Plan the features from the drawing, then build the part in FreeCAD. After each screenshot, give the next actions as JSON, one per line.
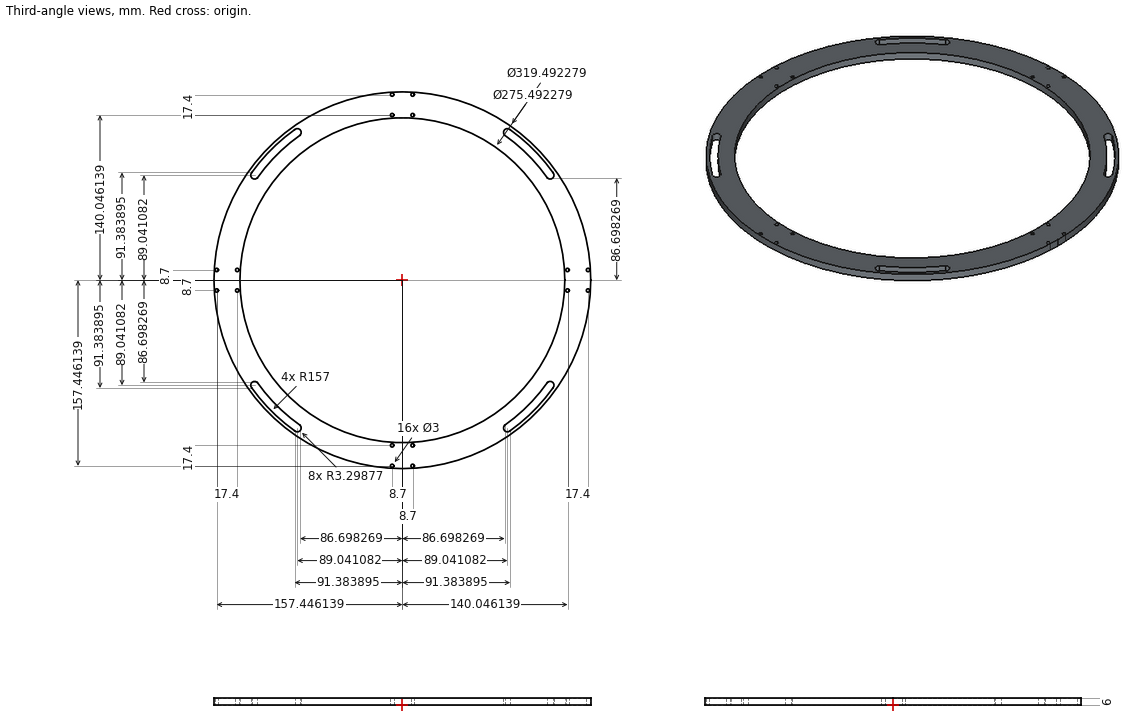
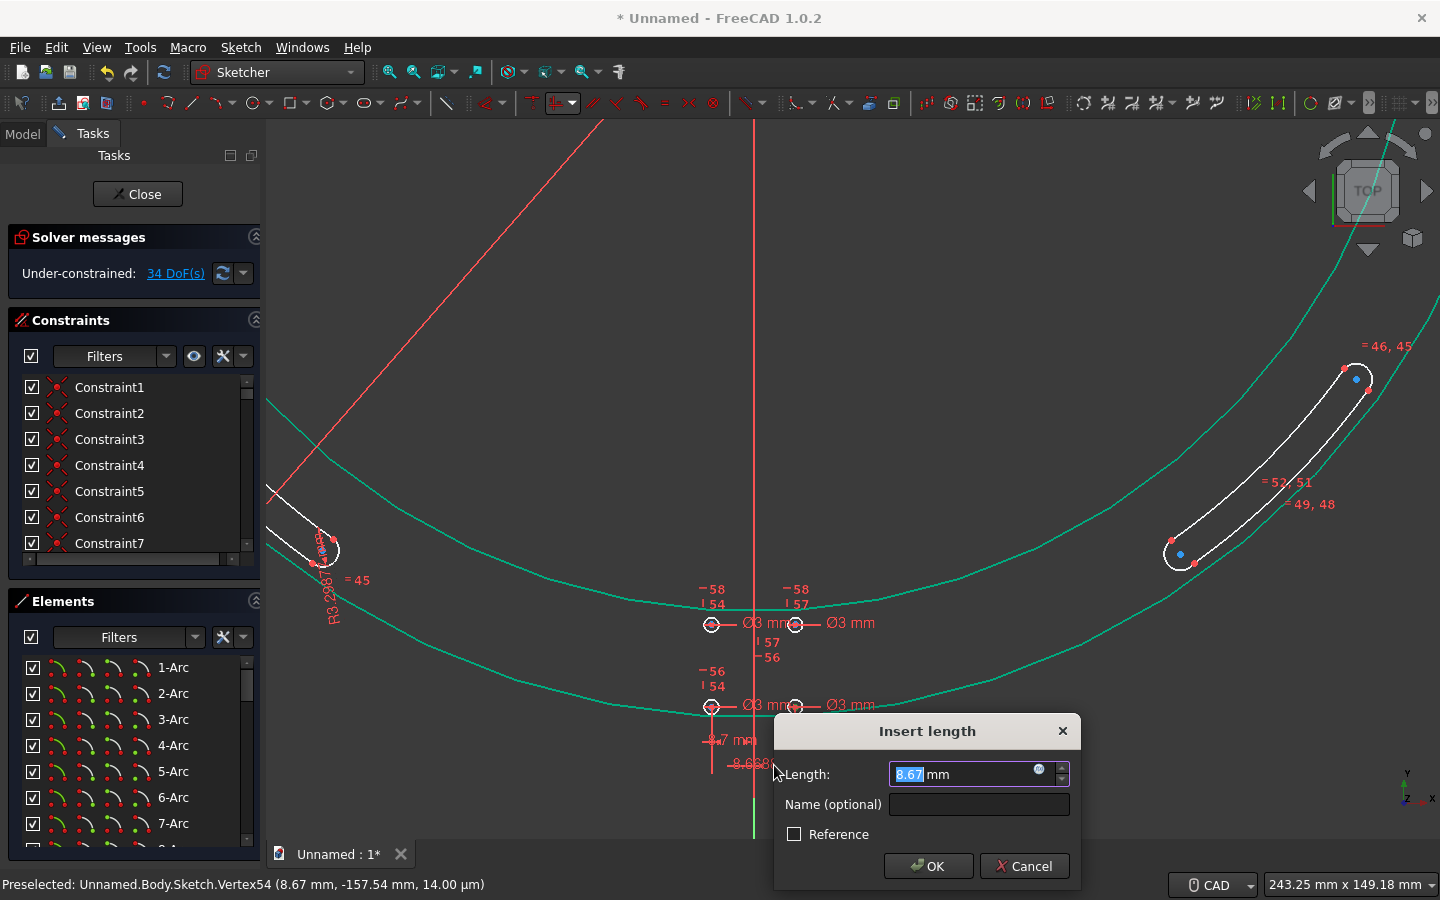
{"action": "type", "text": "8.7"}
{"action": "key", "text": "Return"}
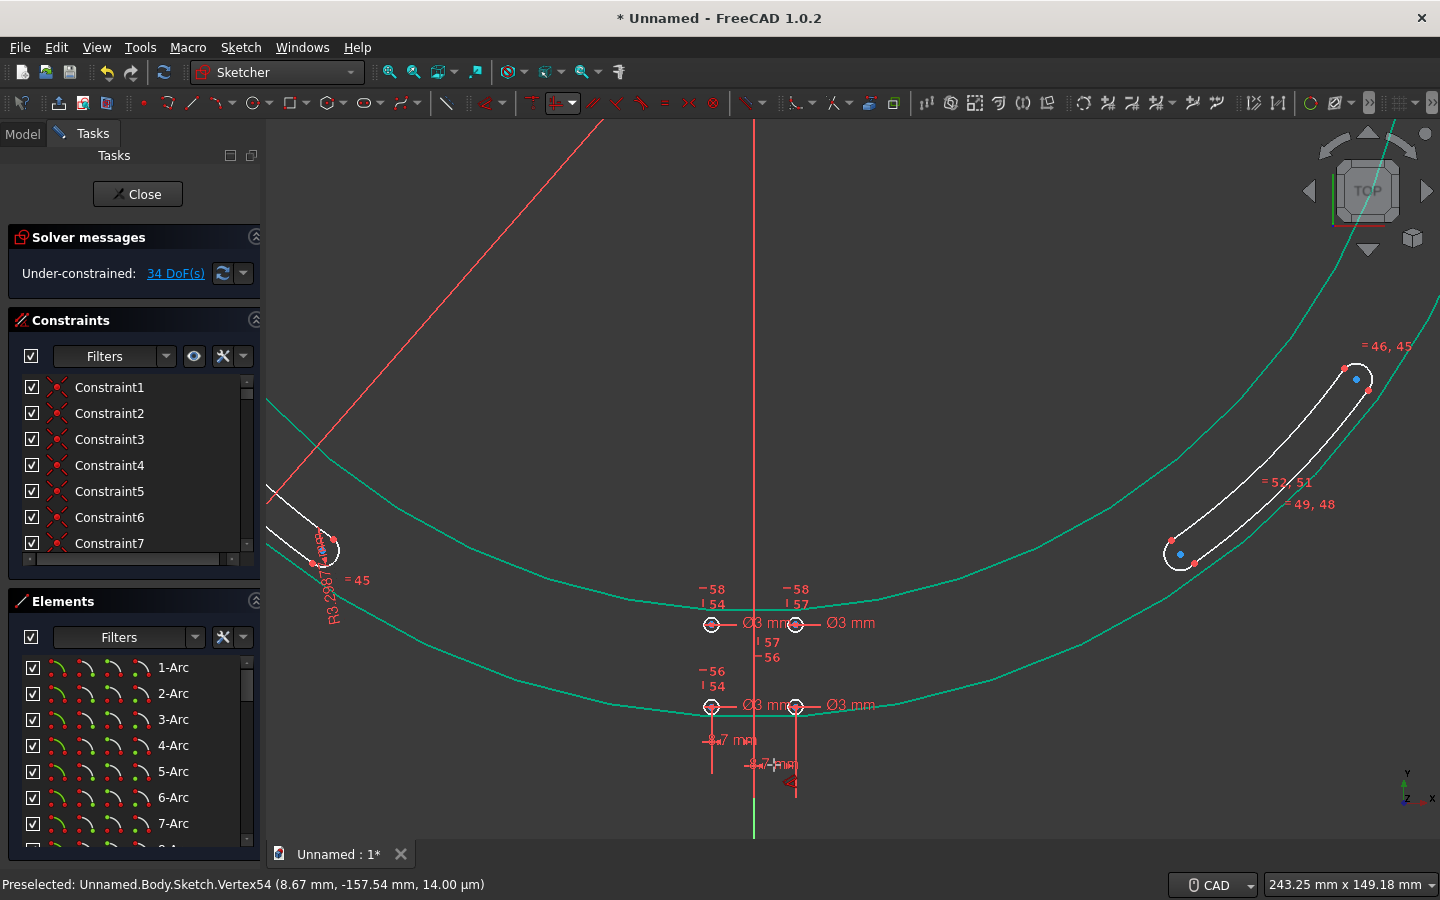
{"action": "scroll", "coordinate": [798, 708], "scroll_direction": "down", "scroll_amount": 6}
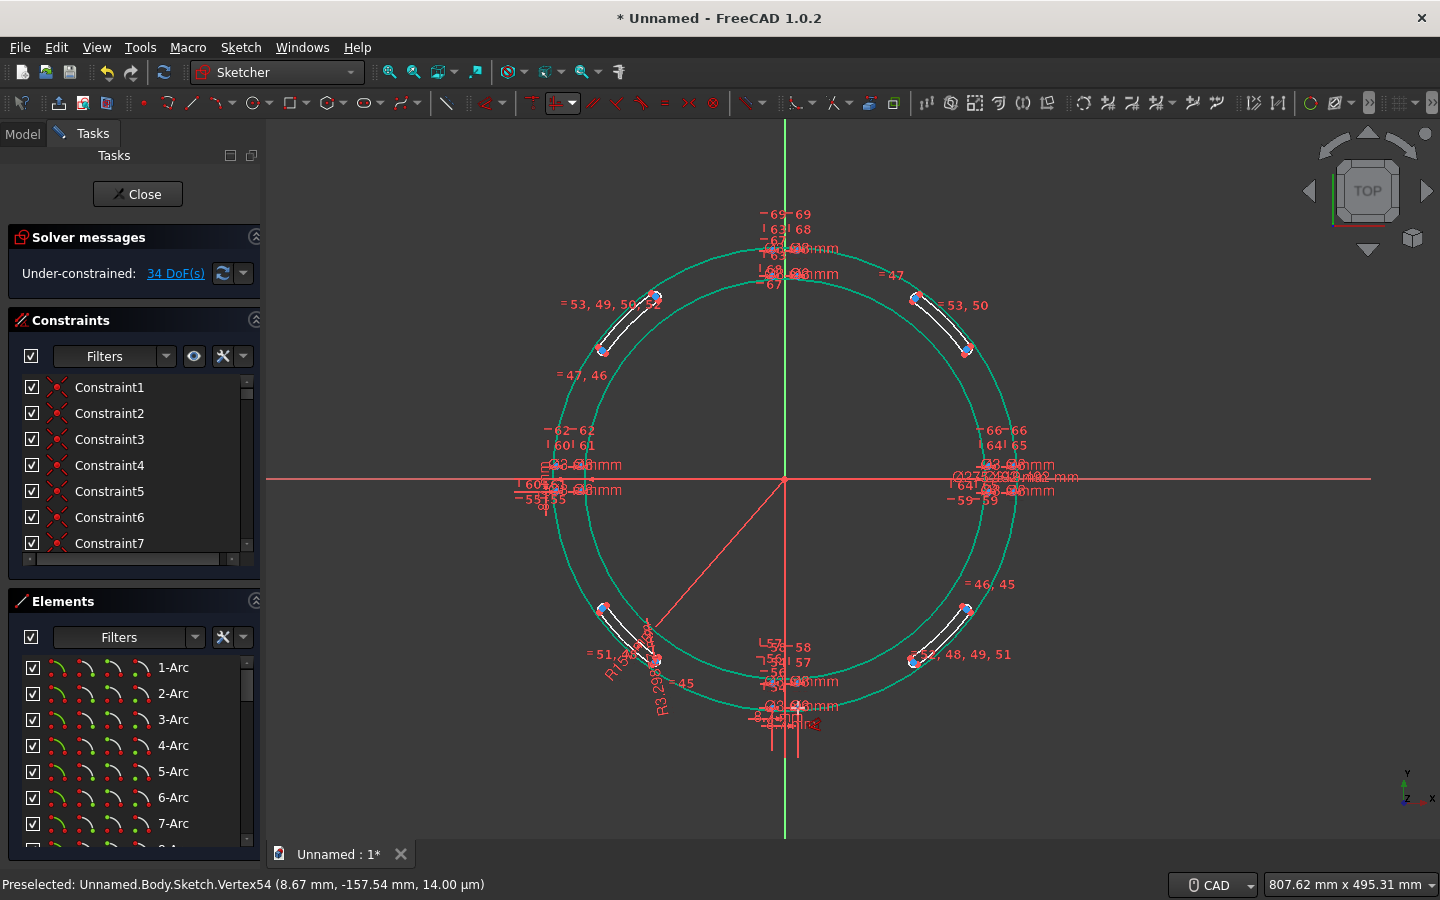
{"action": "scroll", "coordinate": [988, 493], "scroll_direction": "up", "scroll_amount": 6}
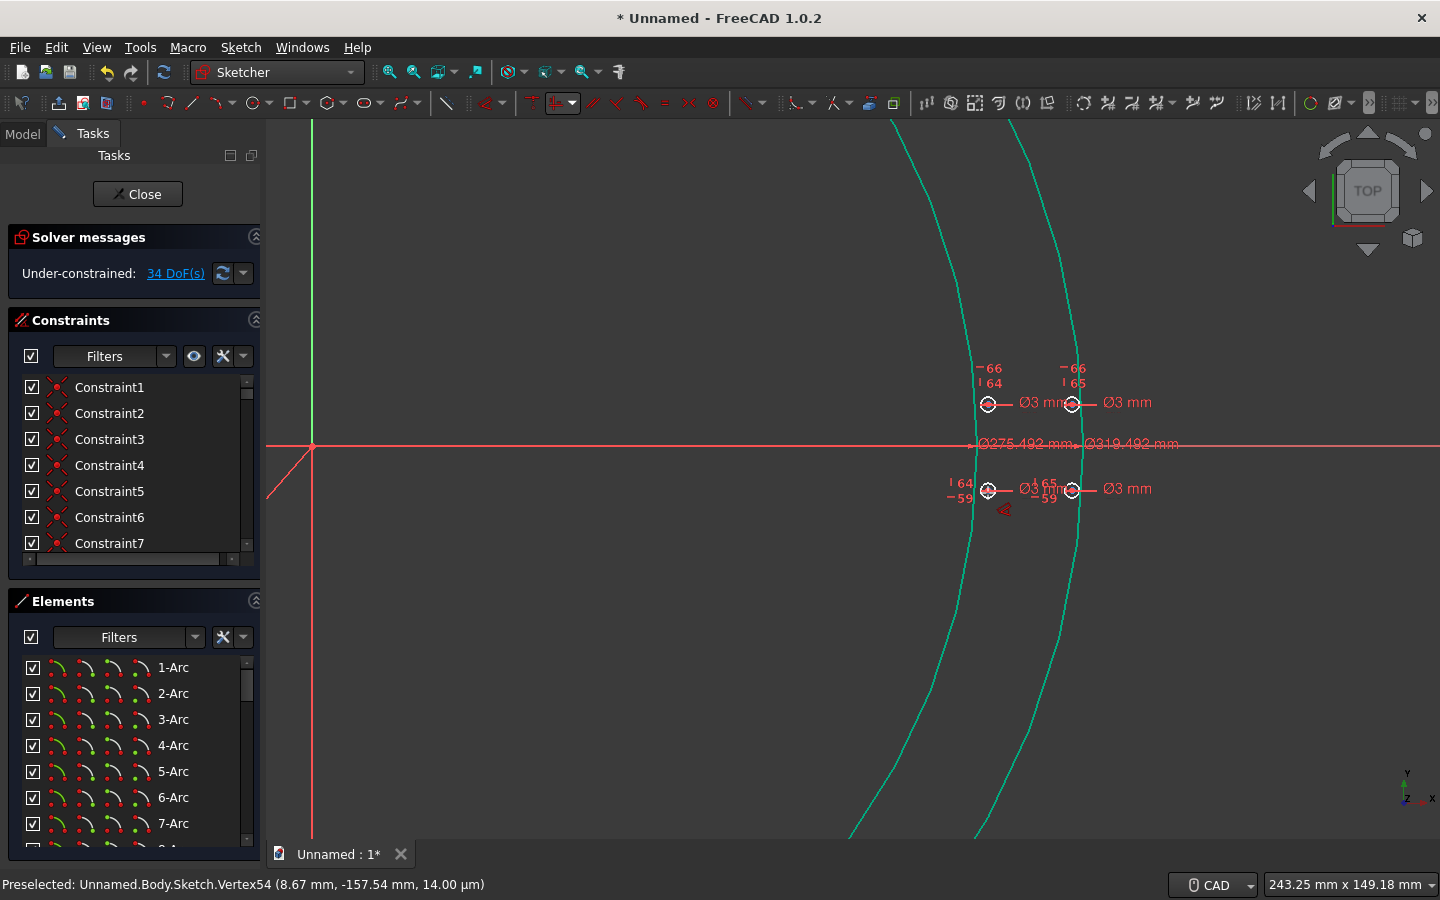
{"action": "left_click", "coordinate": [988, 491]}
{"action": "left_click", "coordinate": [1022, 468]}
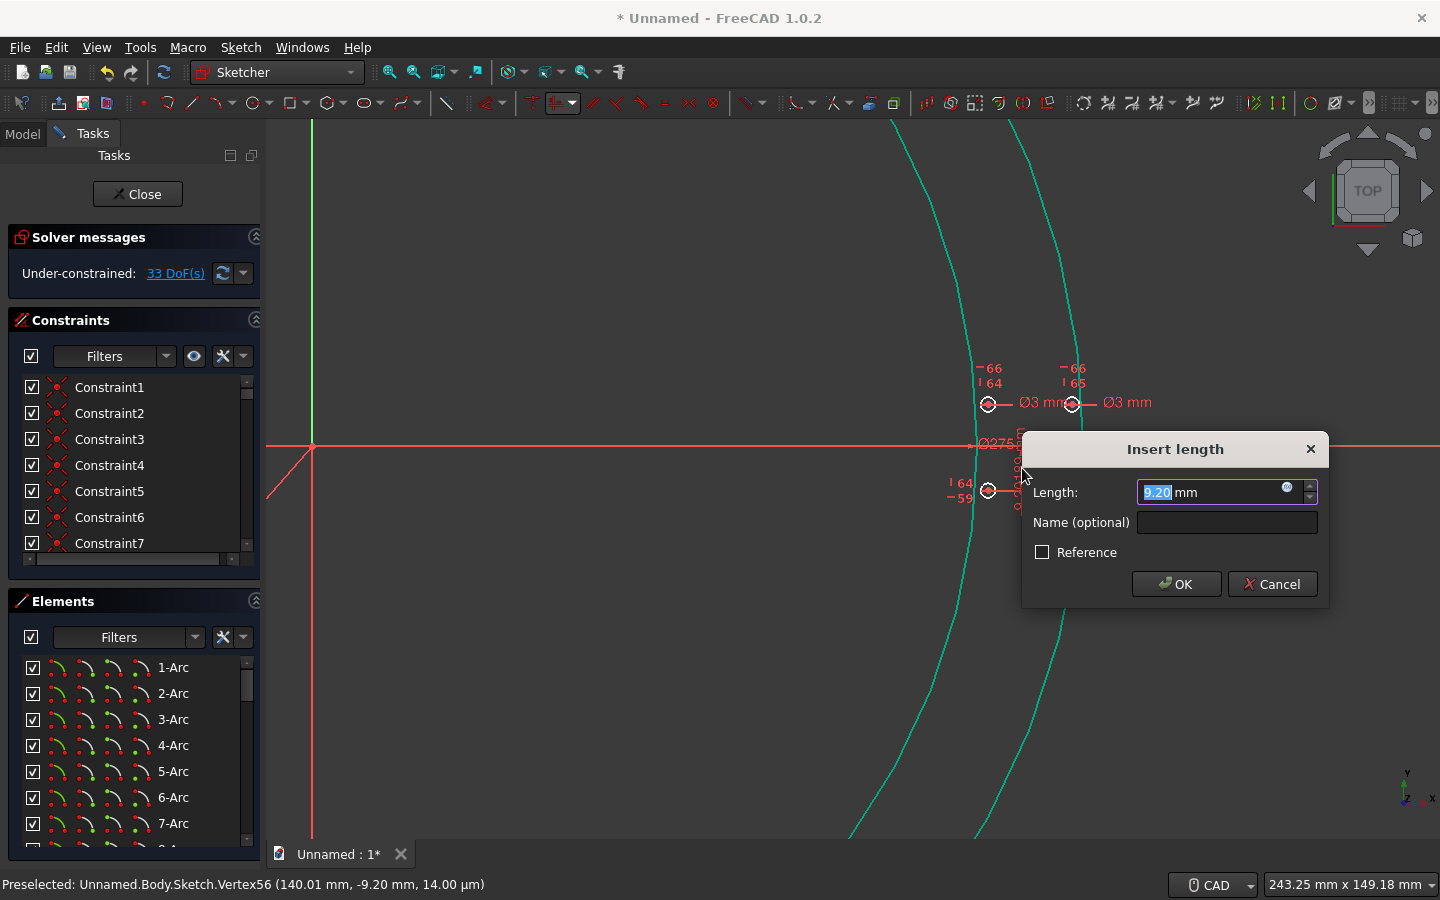
{"action": "type", "text": "8.7"}
{"action": "key", "text": "Return"}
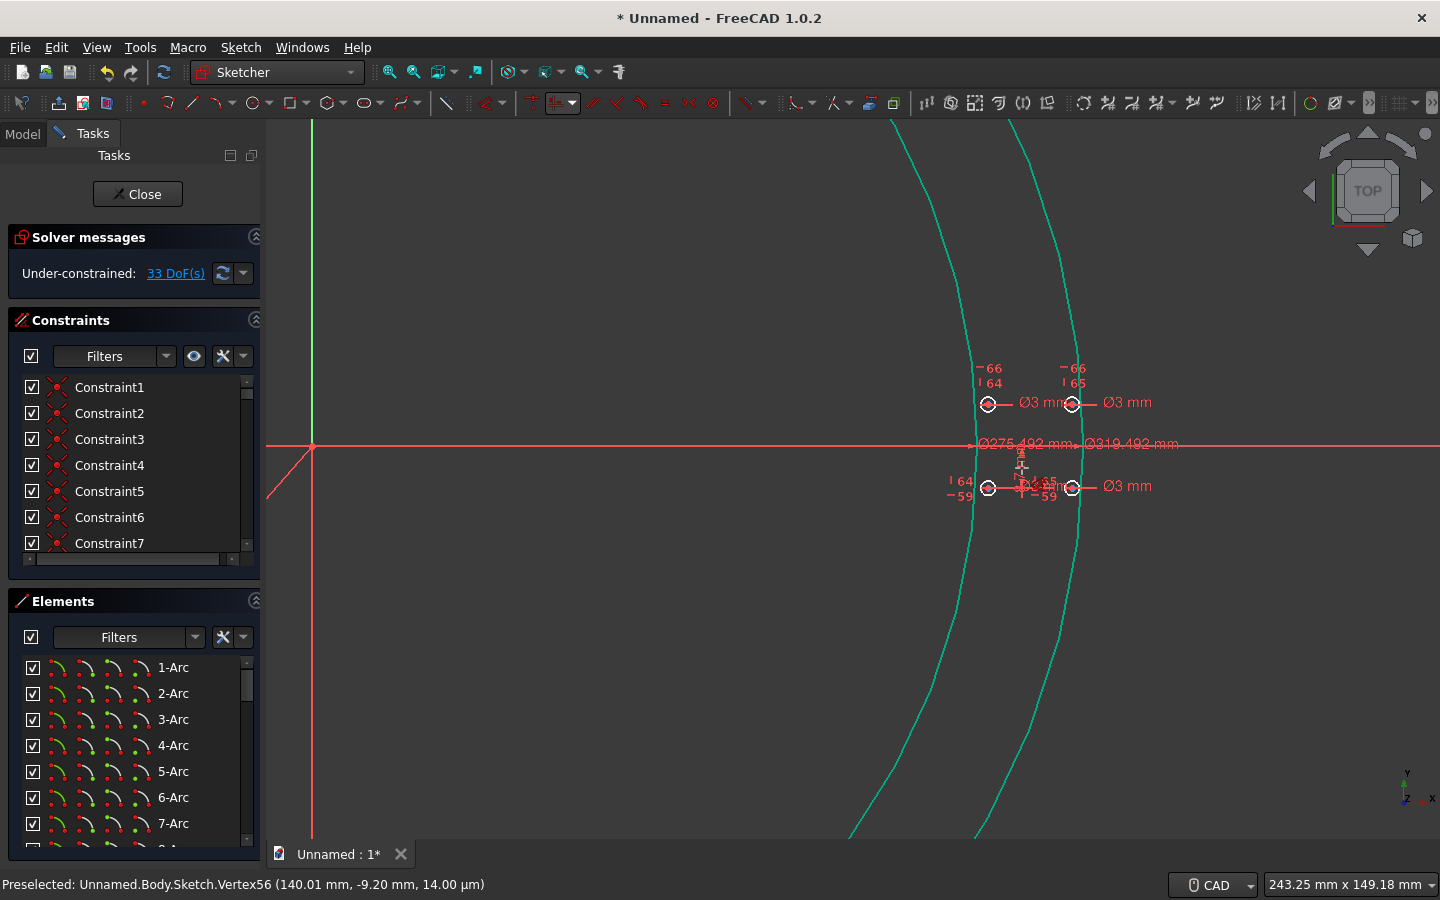
{"action": "scroll", "coordinate": [988, 493], "scroll_direction": "down", "scroll_amount": 6}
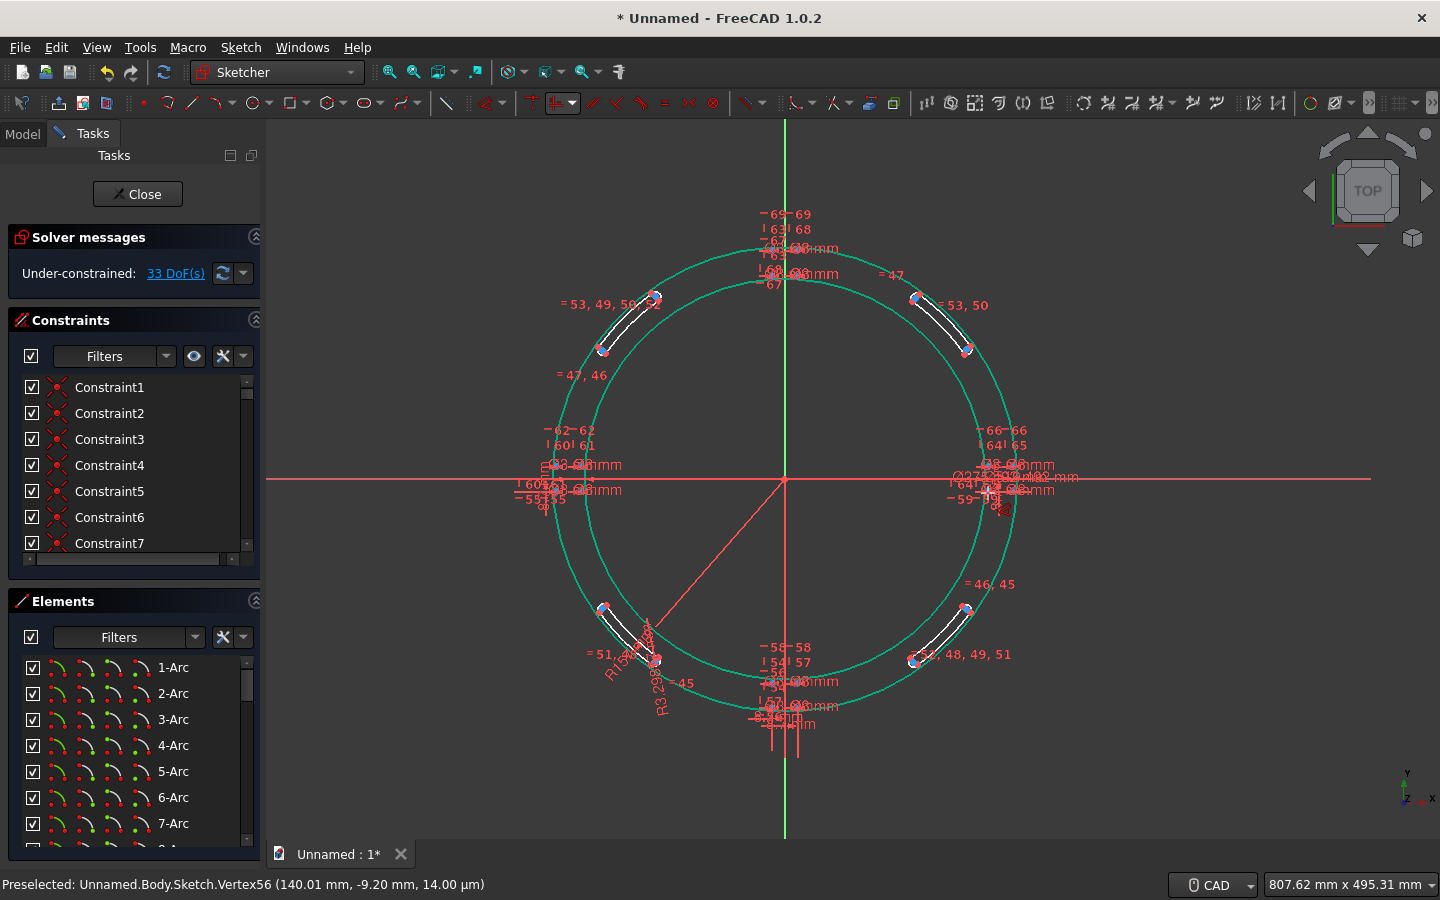
{"action": "scroll", "coordinate": [556, 467], "scroll_direction": "up", "scroll_amount": 6}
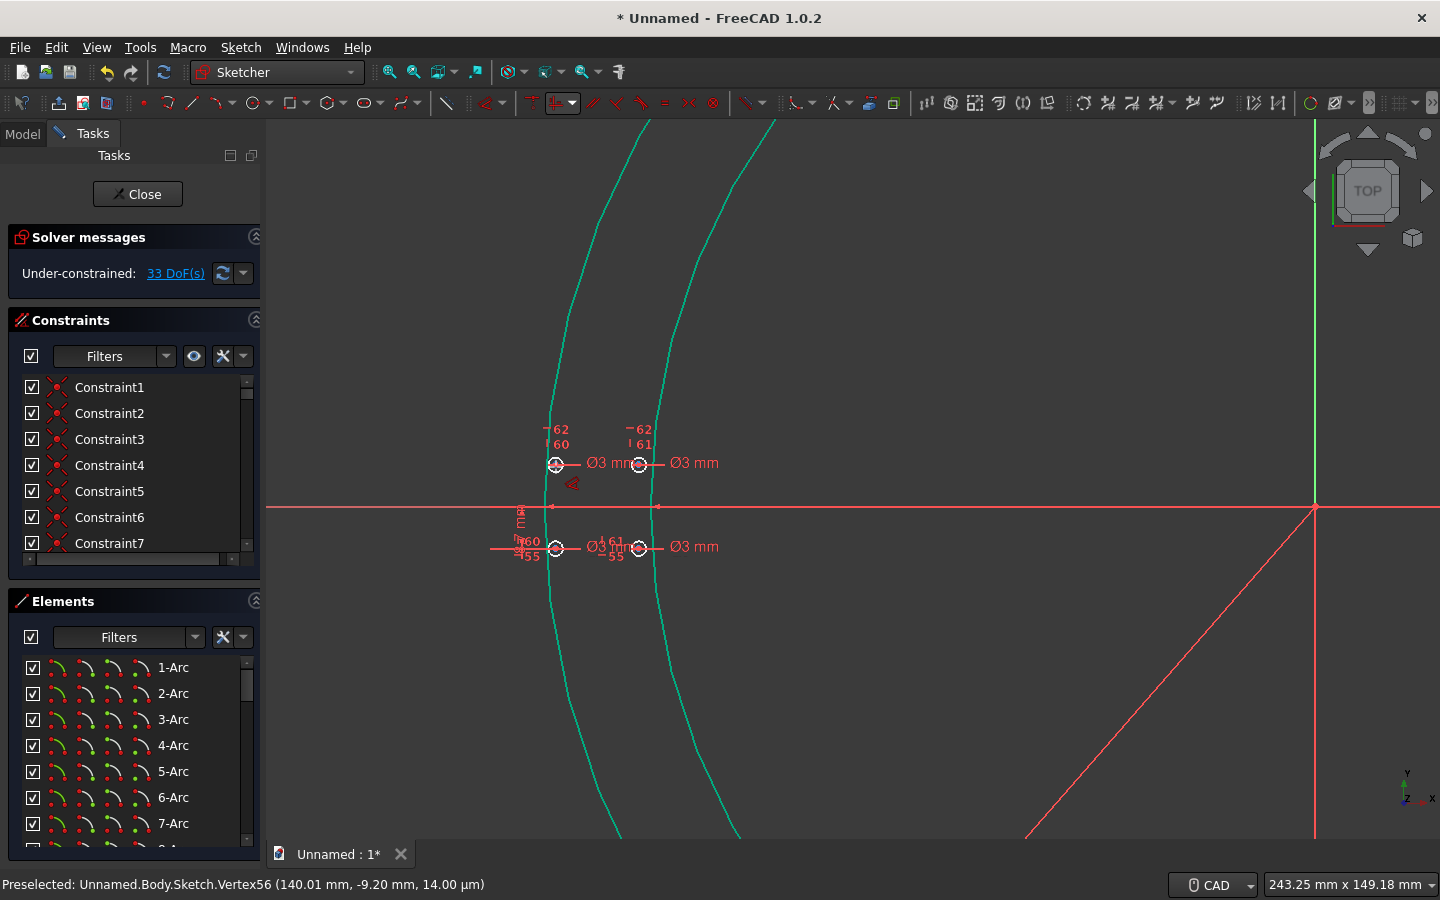
{"action": "left_click", "coordinate": [556, 465]}
{"action": "left_click", "coordinate": [522, 486]}